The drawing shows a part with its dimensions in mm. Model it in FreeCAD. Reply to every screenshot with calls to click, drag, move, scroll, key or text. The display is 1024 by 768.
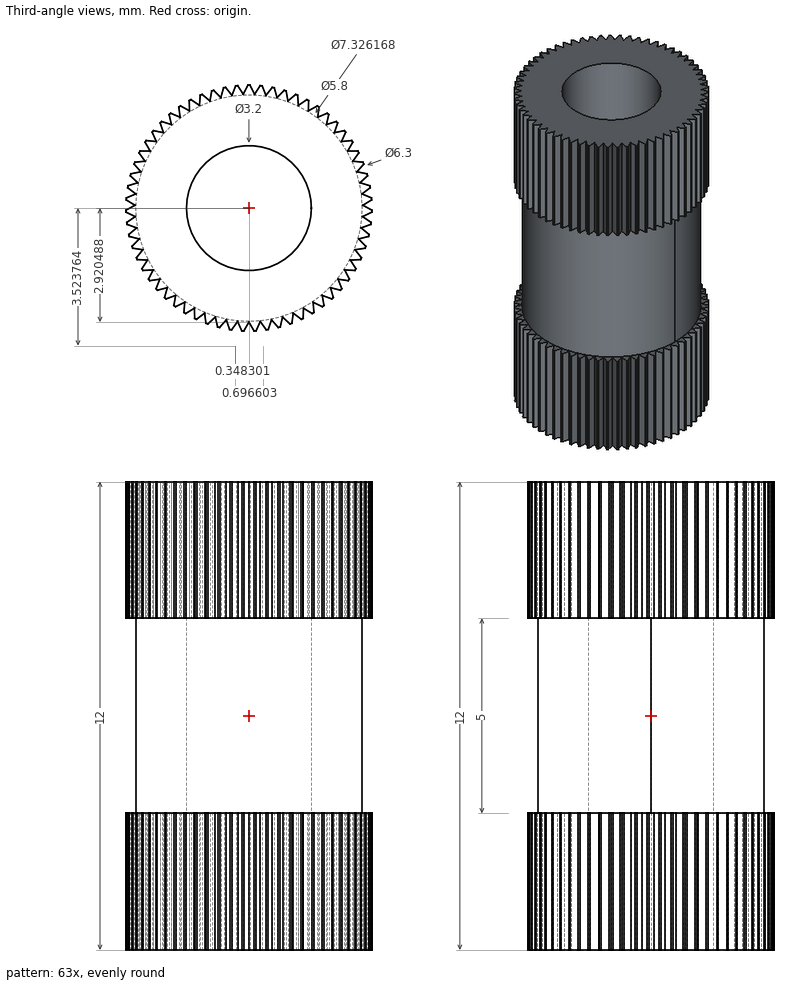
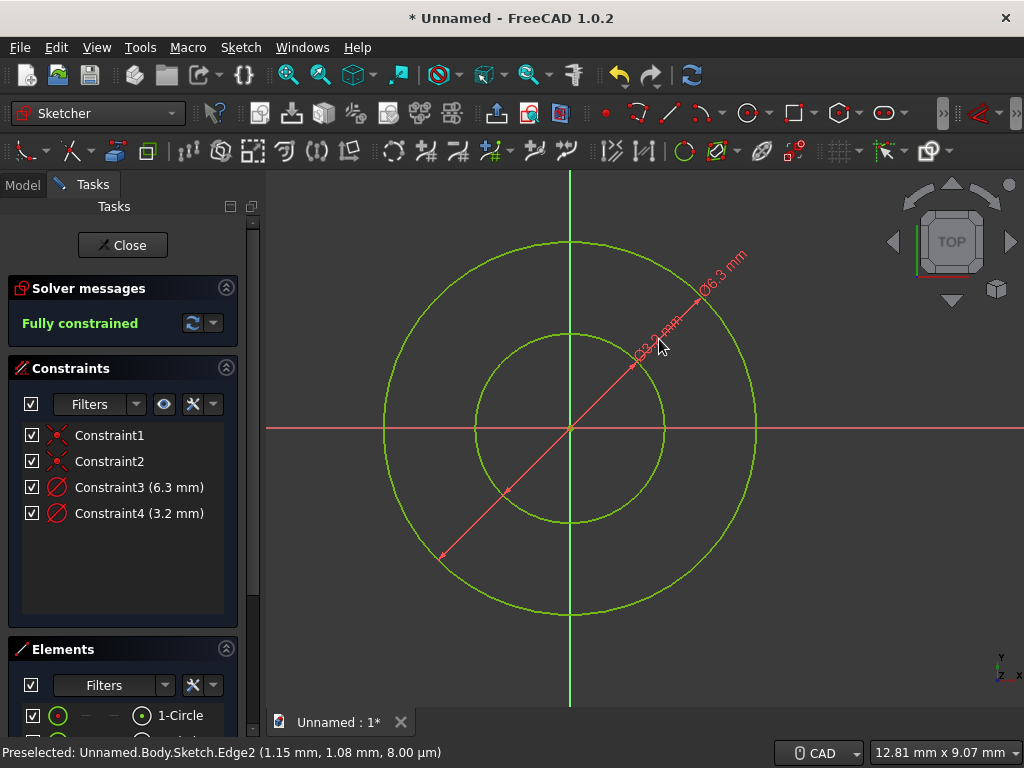
click(123, 245)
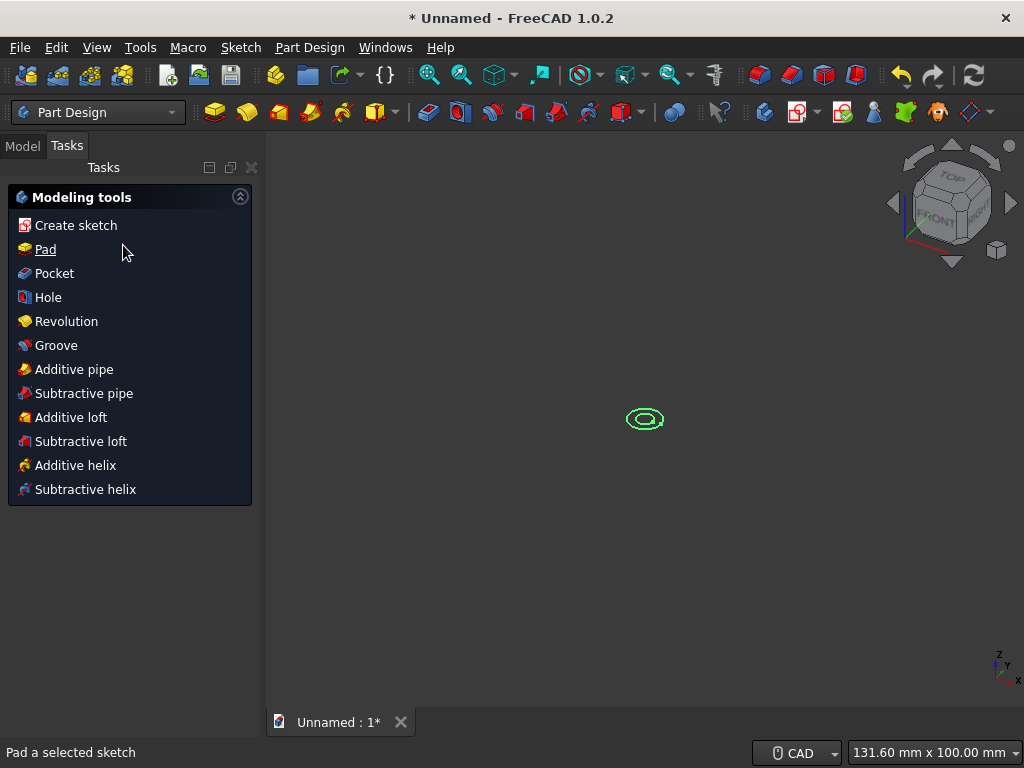
click(216, 112)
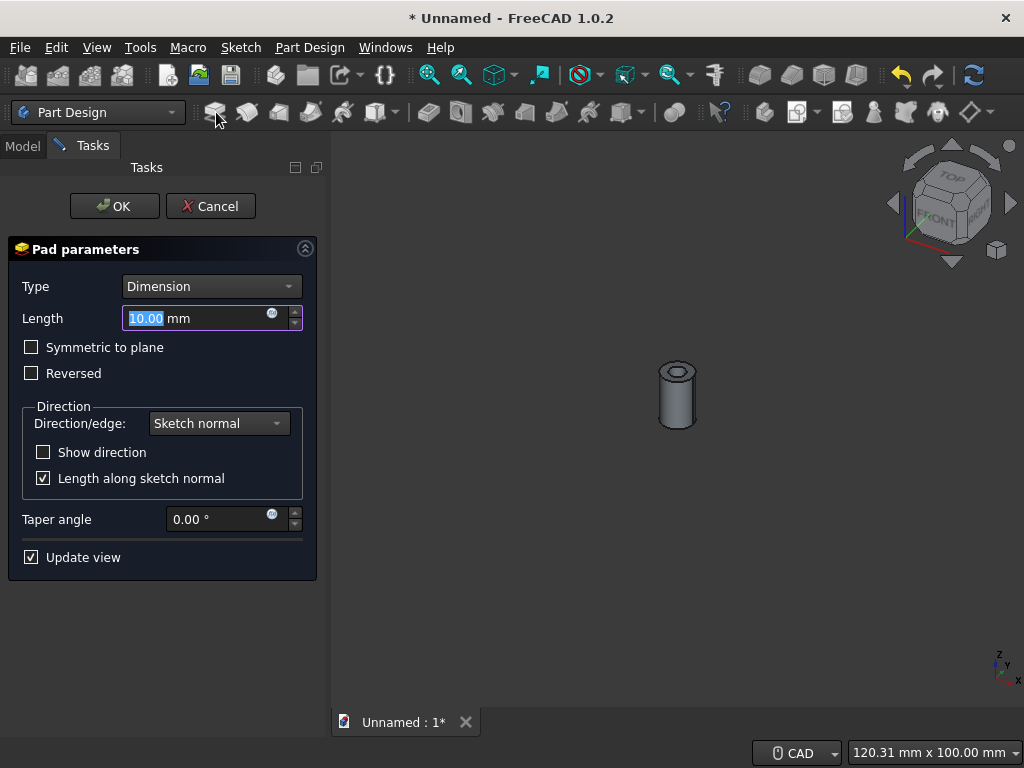
text(12)
key(Tab)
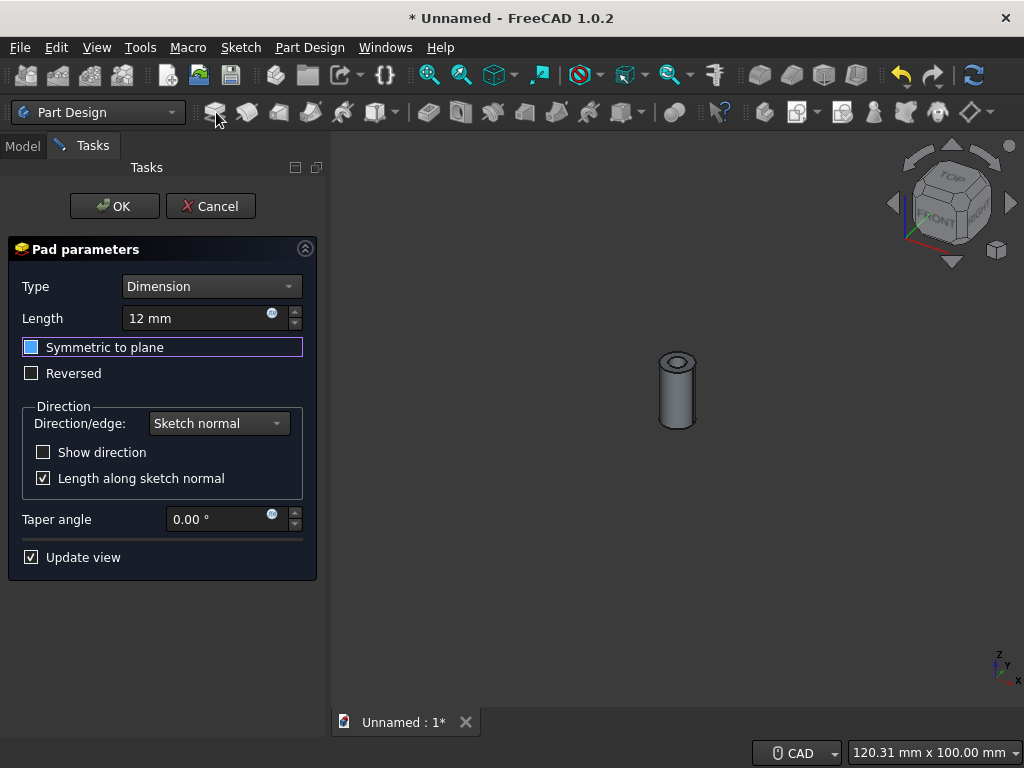
click(30, 347)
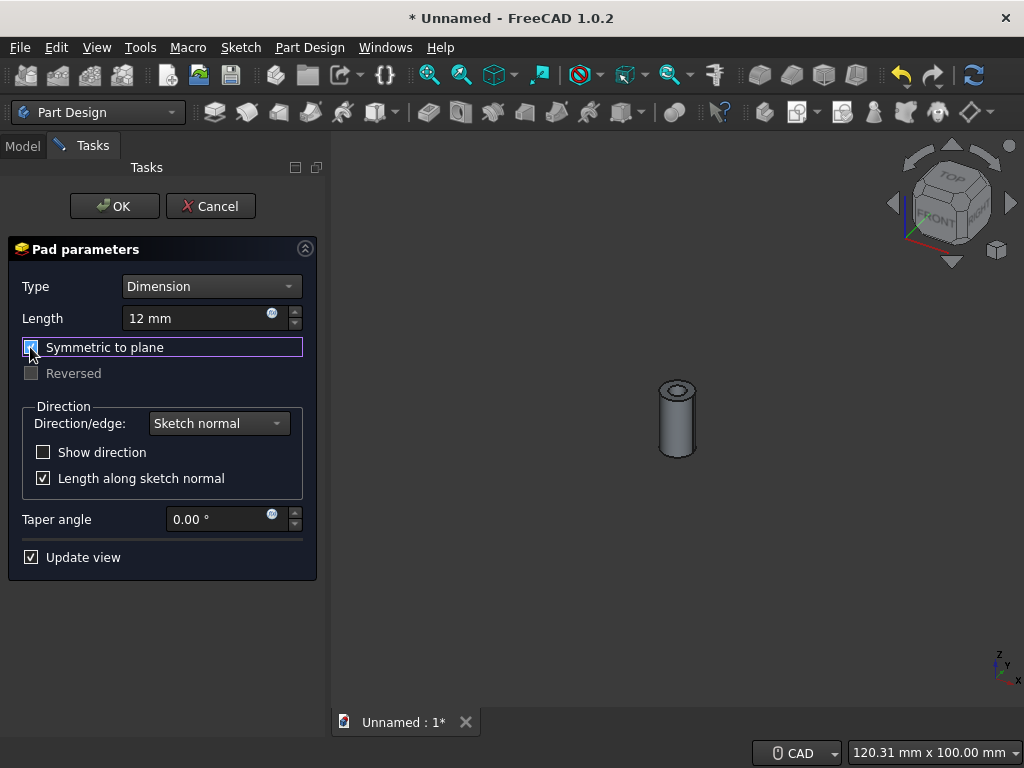
click(115, 206)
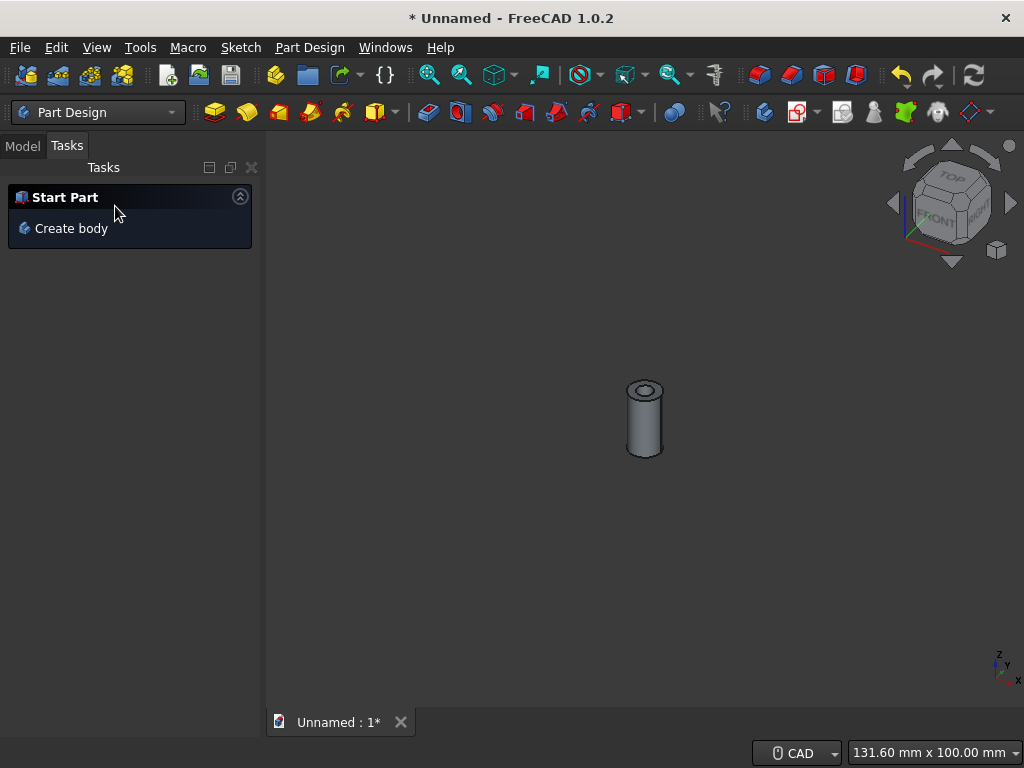
click(430, 76)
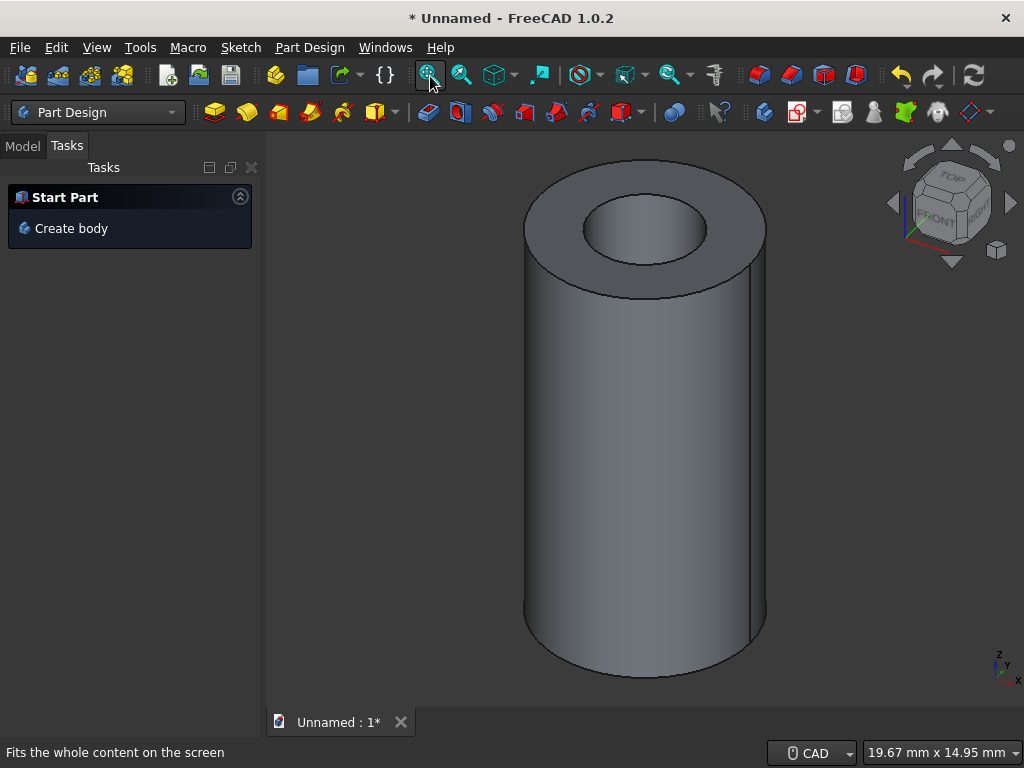
click(550, 243)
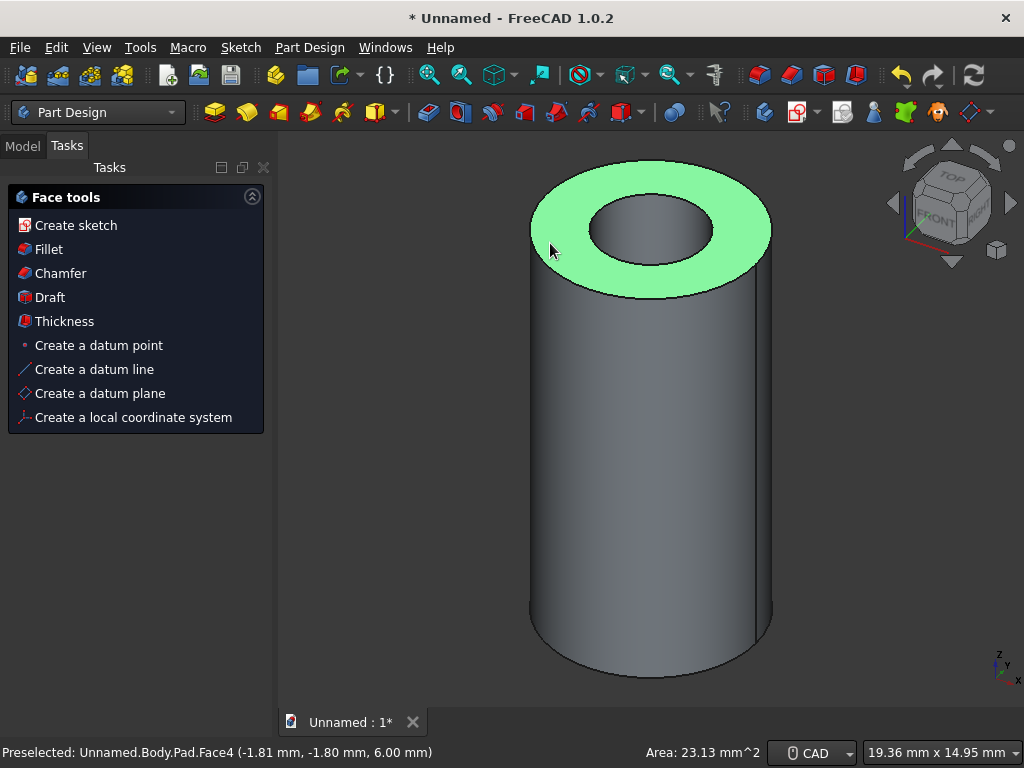
click(798, 112)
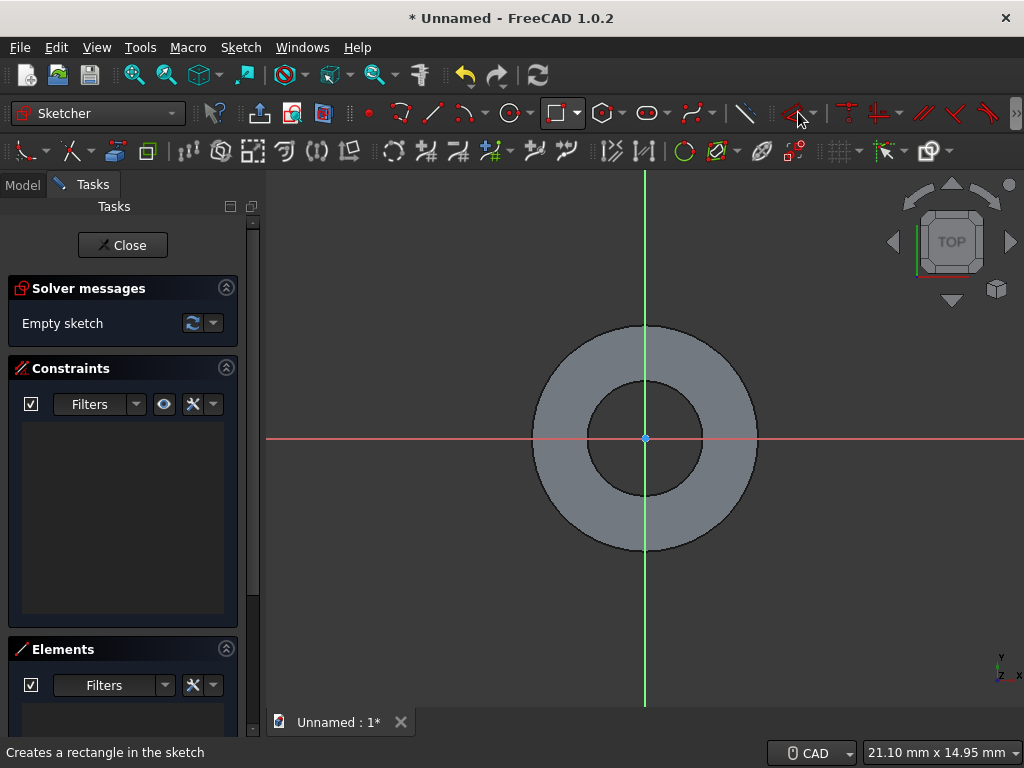
scroll(649, 562, up, 14)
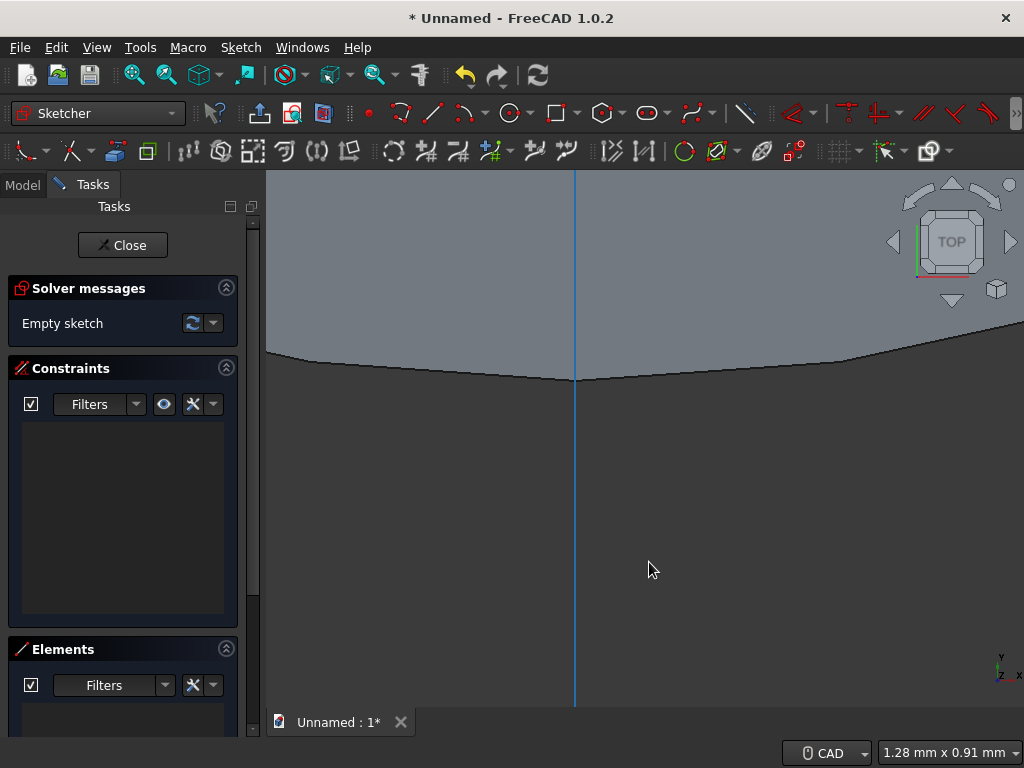
click(402, 114)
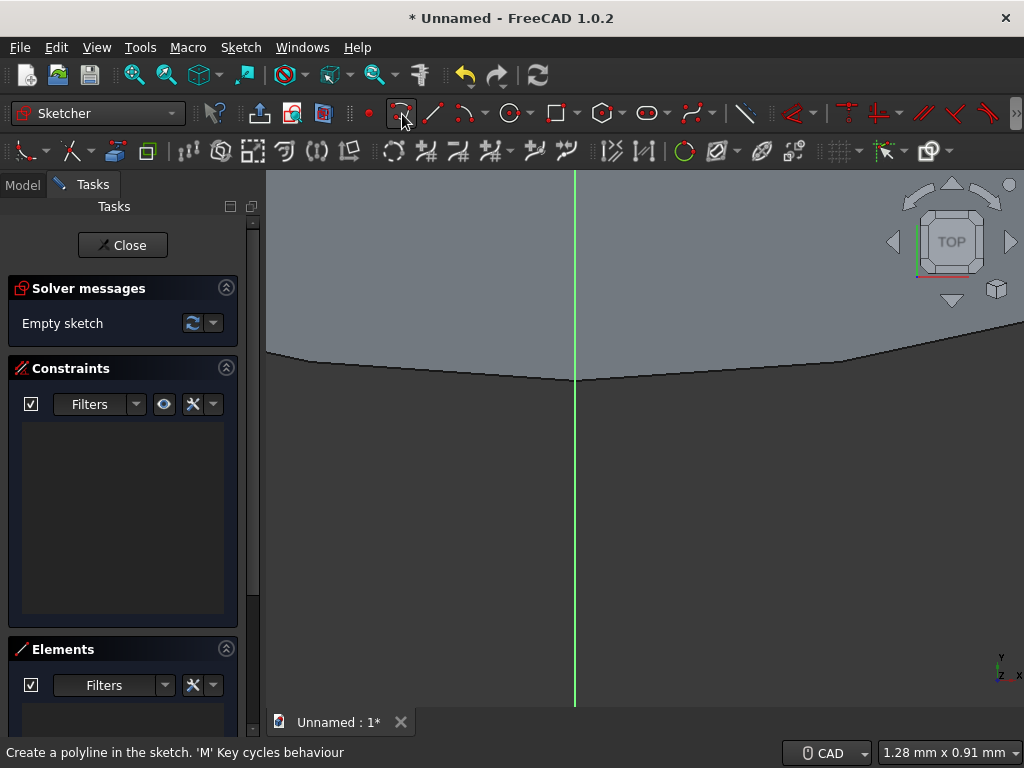
click(575, 245)
click(370, 602)
click(781, 602)
click(575, 246)
key(Escape)
key(Escape)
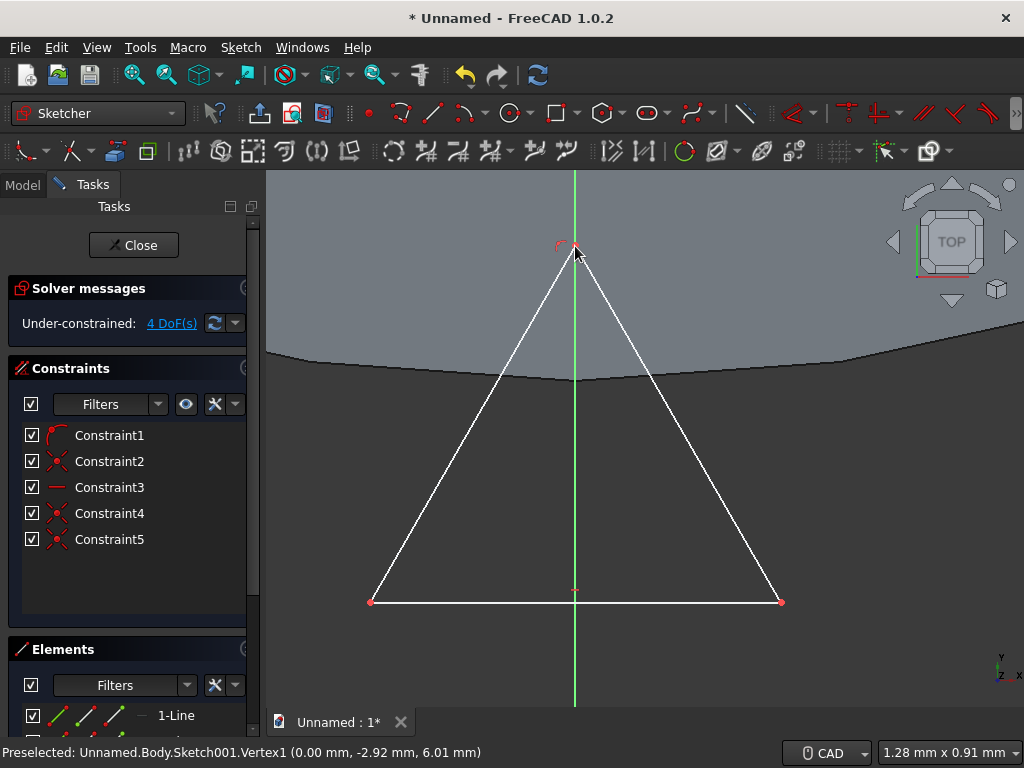
click(792, 114)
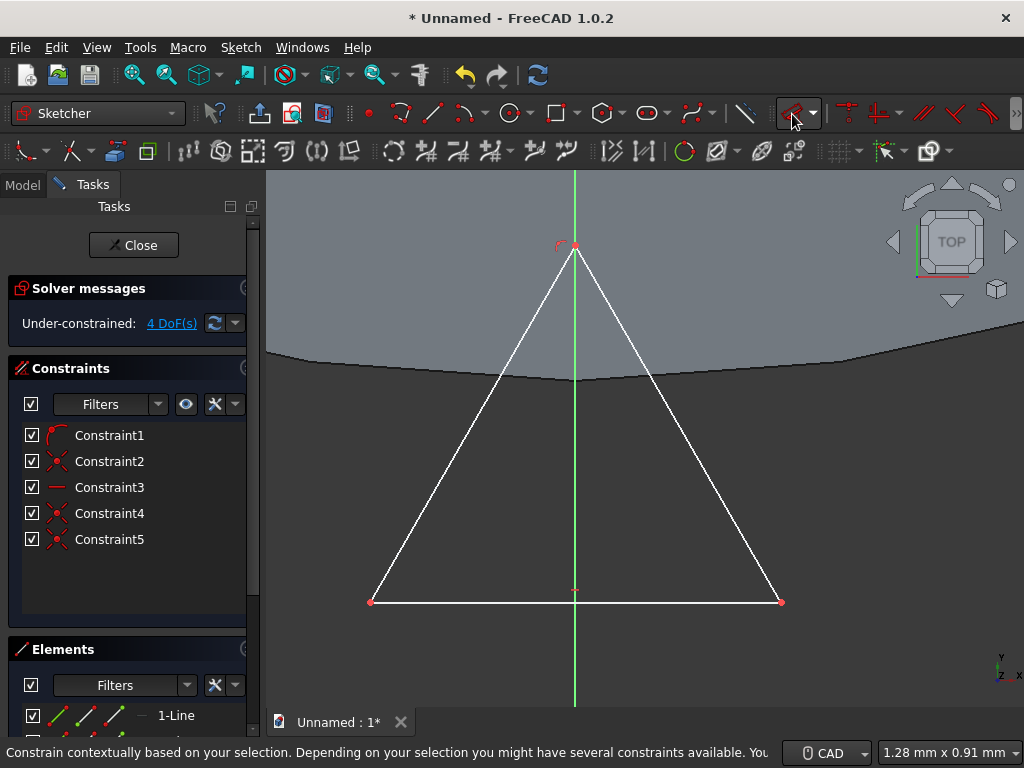
click(493, 603)
click(481, 637)